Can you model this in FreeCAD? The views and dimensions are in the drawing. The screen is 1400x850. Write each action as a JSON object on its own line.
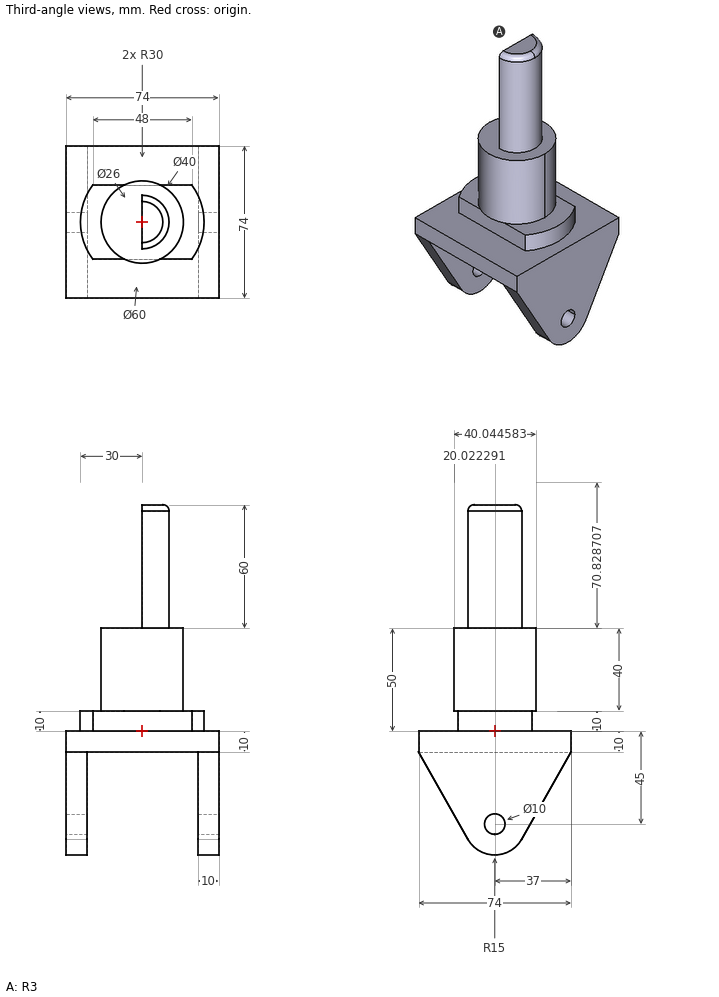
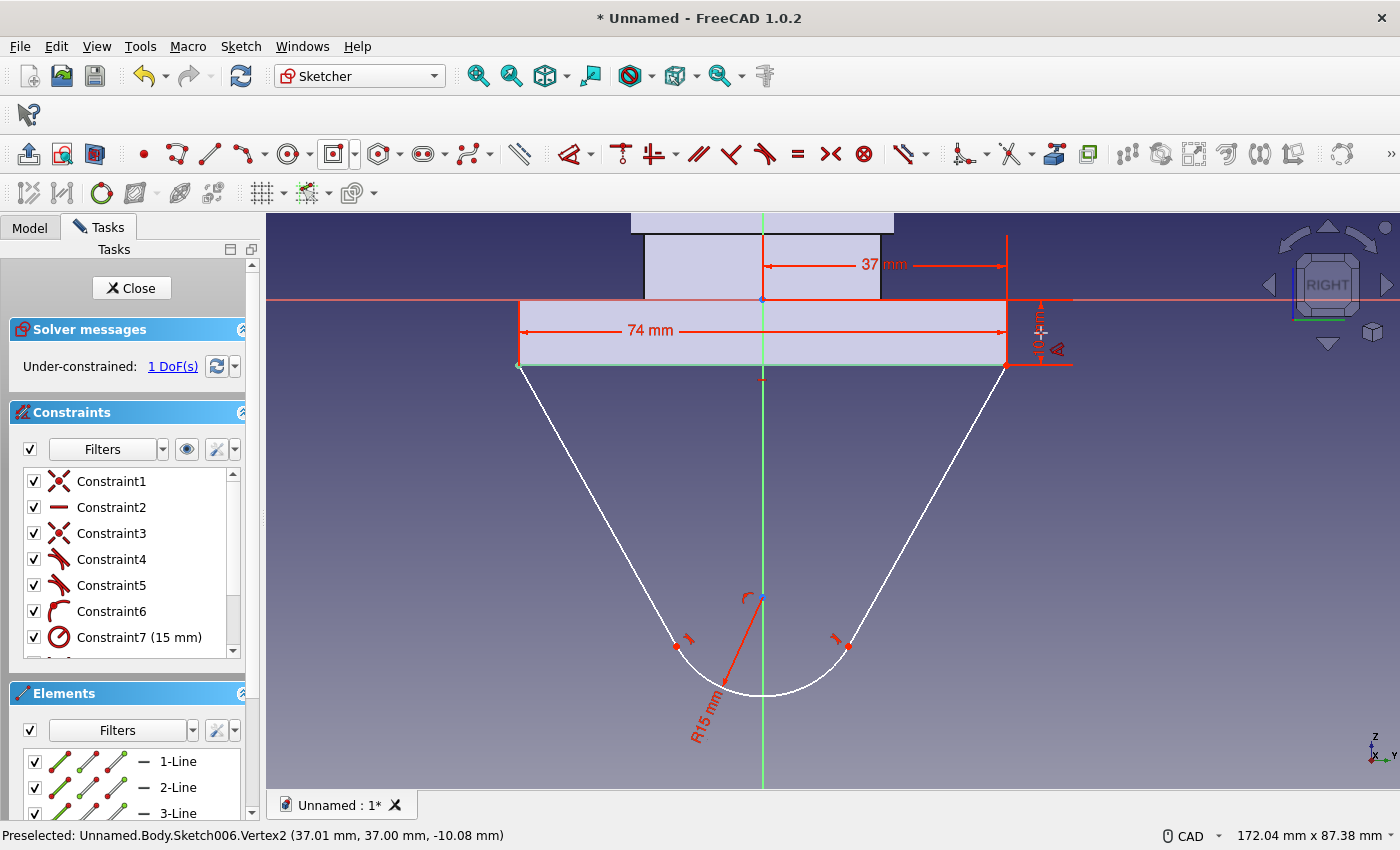
{"action": "left_click", "coordinate": [763, 598]}
{"action": "left_click", "coordinate": [797, 449]}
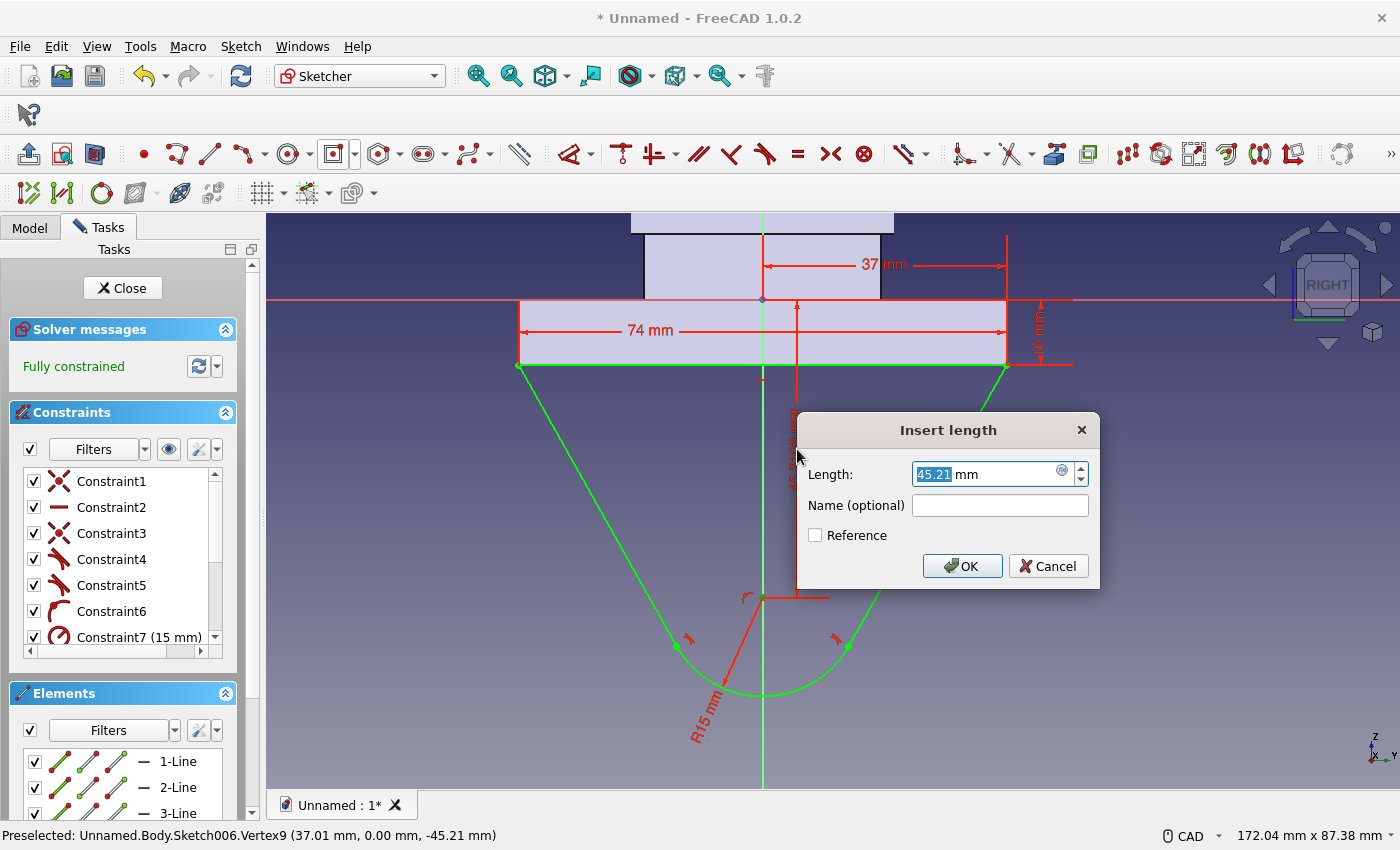
{"action": "type", "text": "45"}
{"action": "key", "text": "Return"}
{"action": "key", "text": "Escape"}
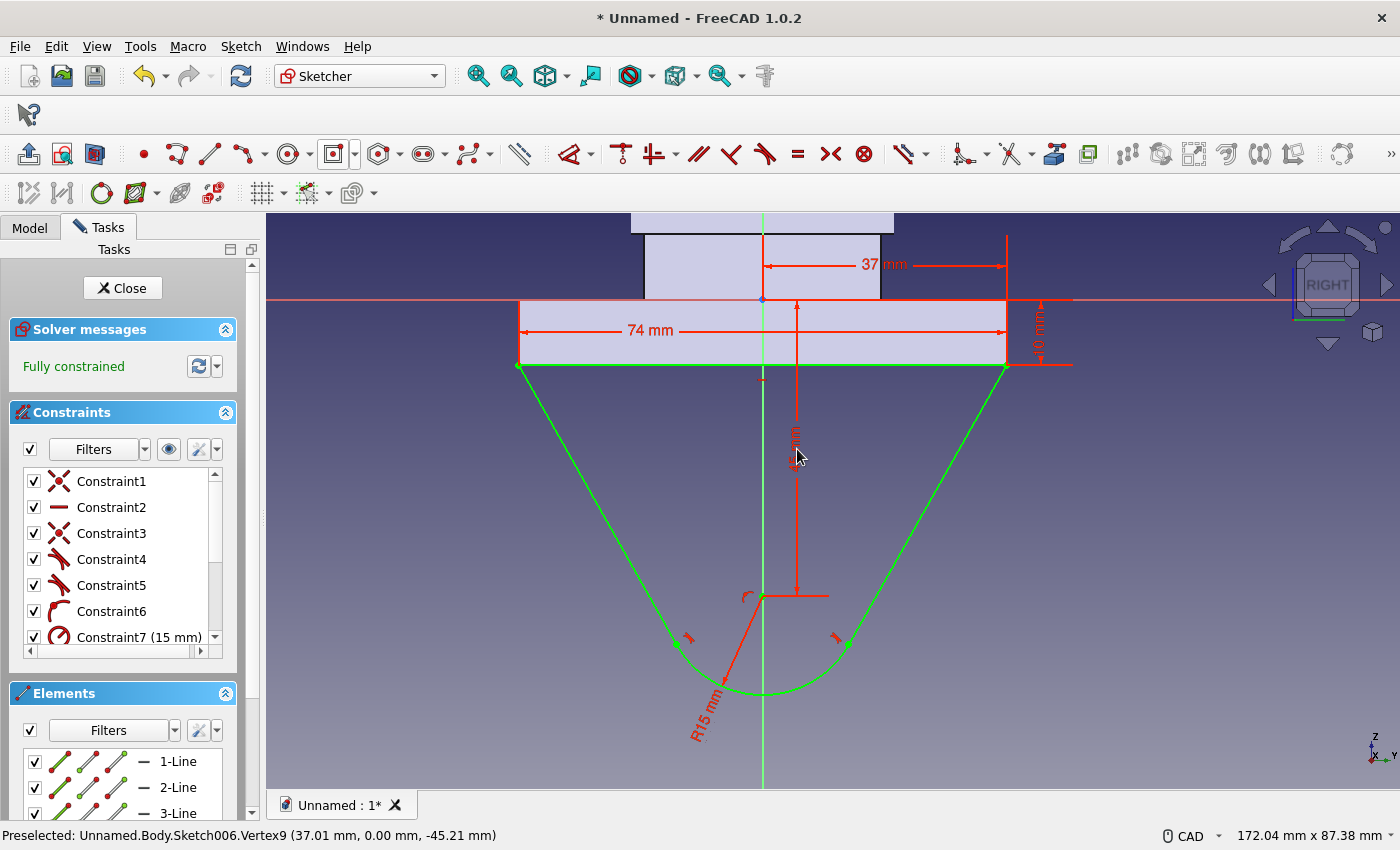
{"action": "left_click", "coordinate": [123, 288]}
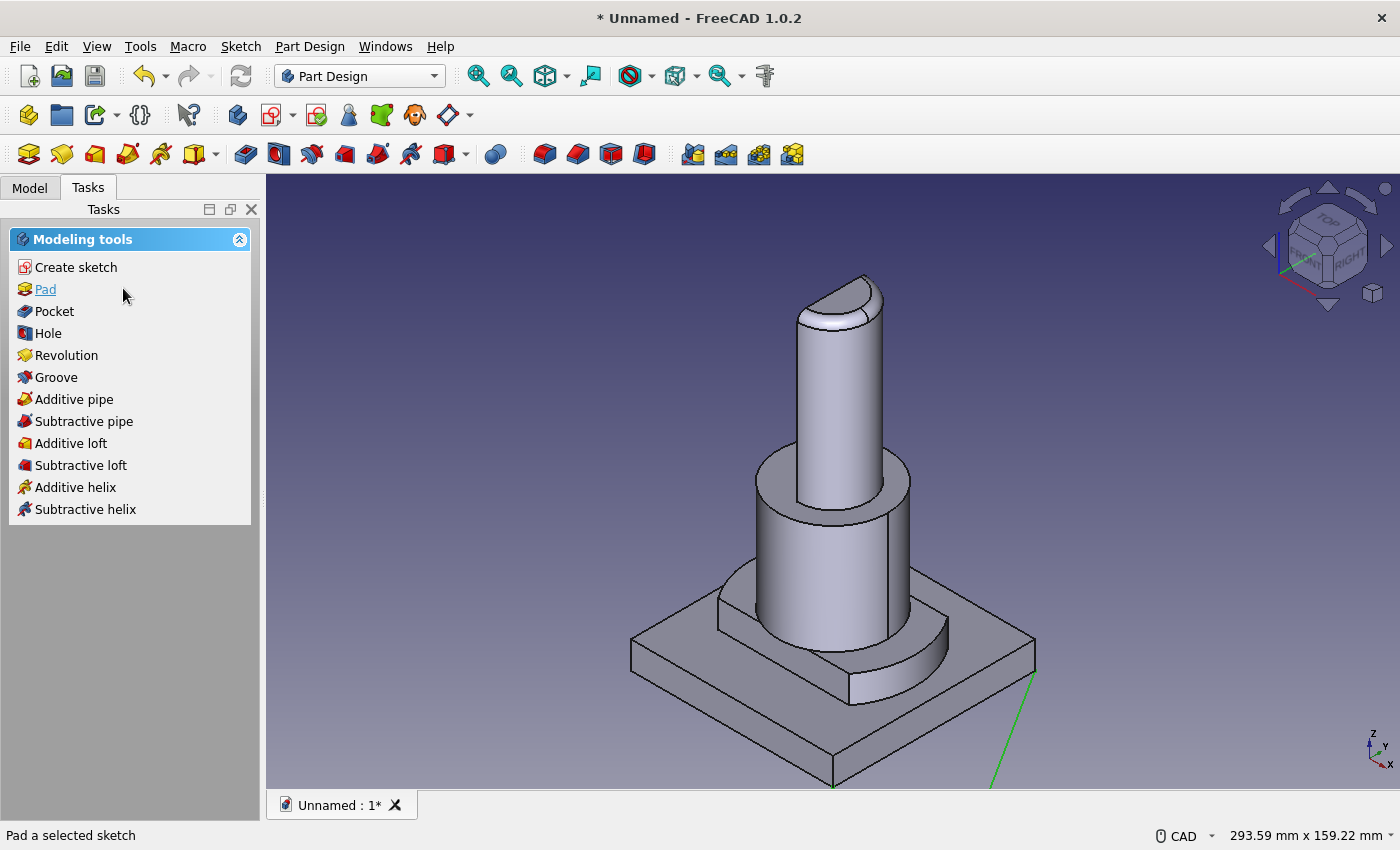
{"action": "left_click", "coordinate": [29, 154]}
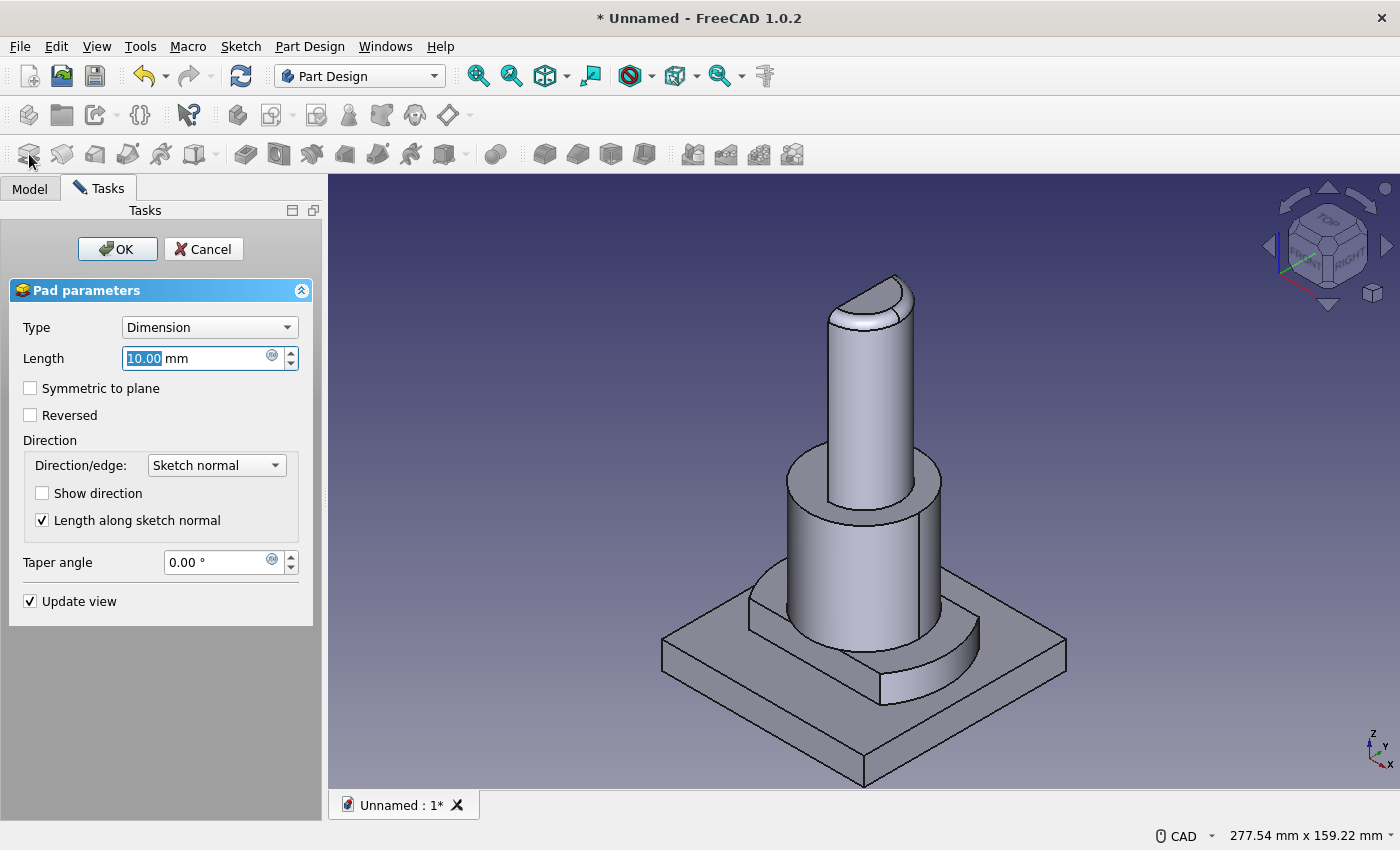
{"action": "type", "text": "10"}
{"action": "key", "text": "Tab"}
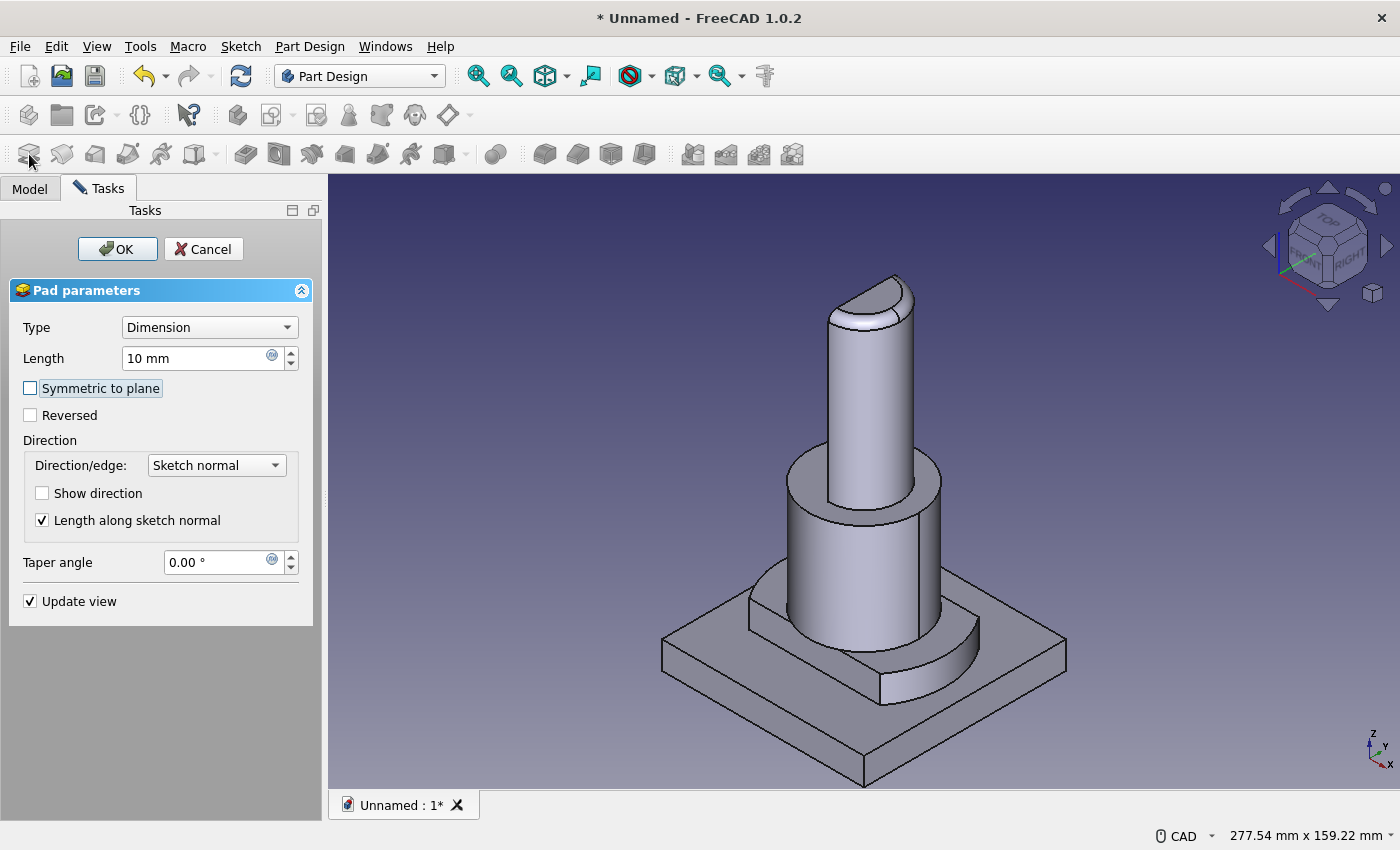
{"action": "left_click", "coordinate": [31, 415]}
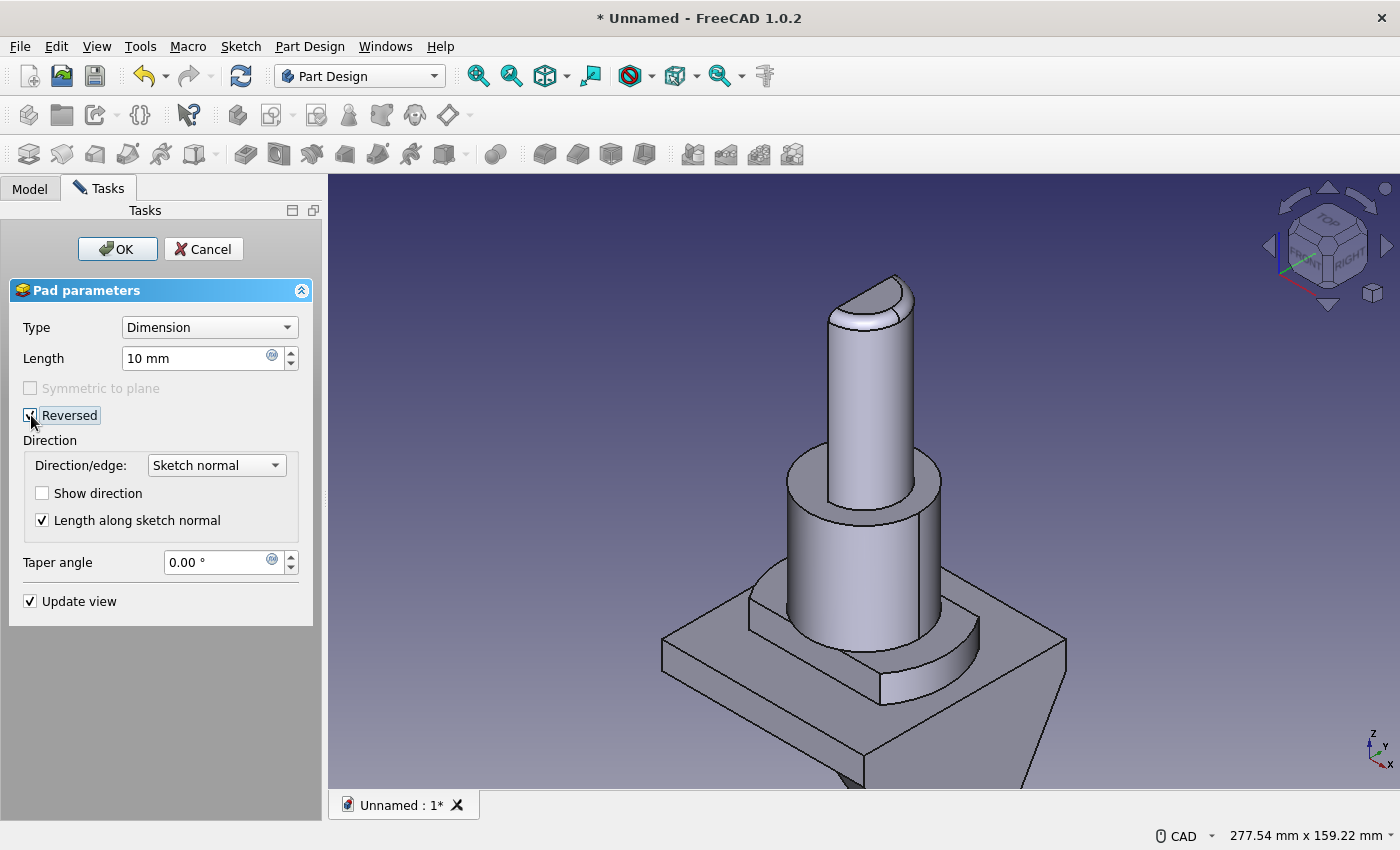
{"action": "left_click", "coordinate": [118, 249]}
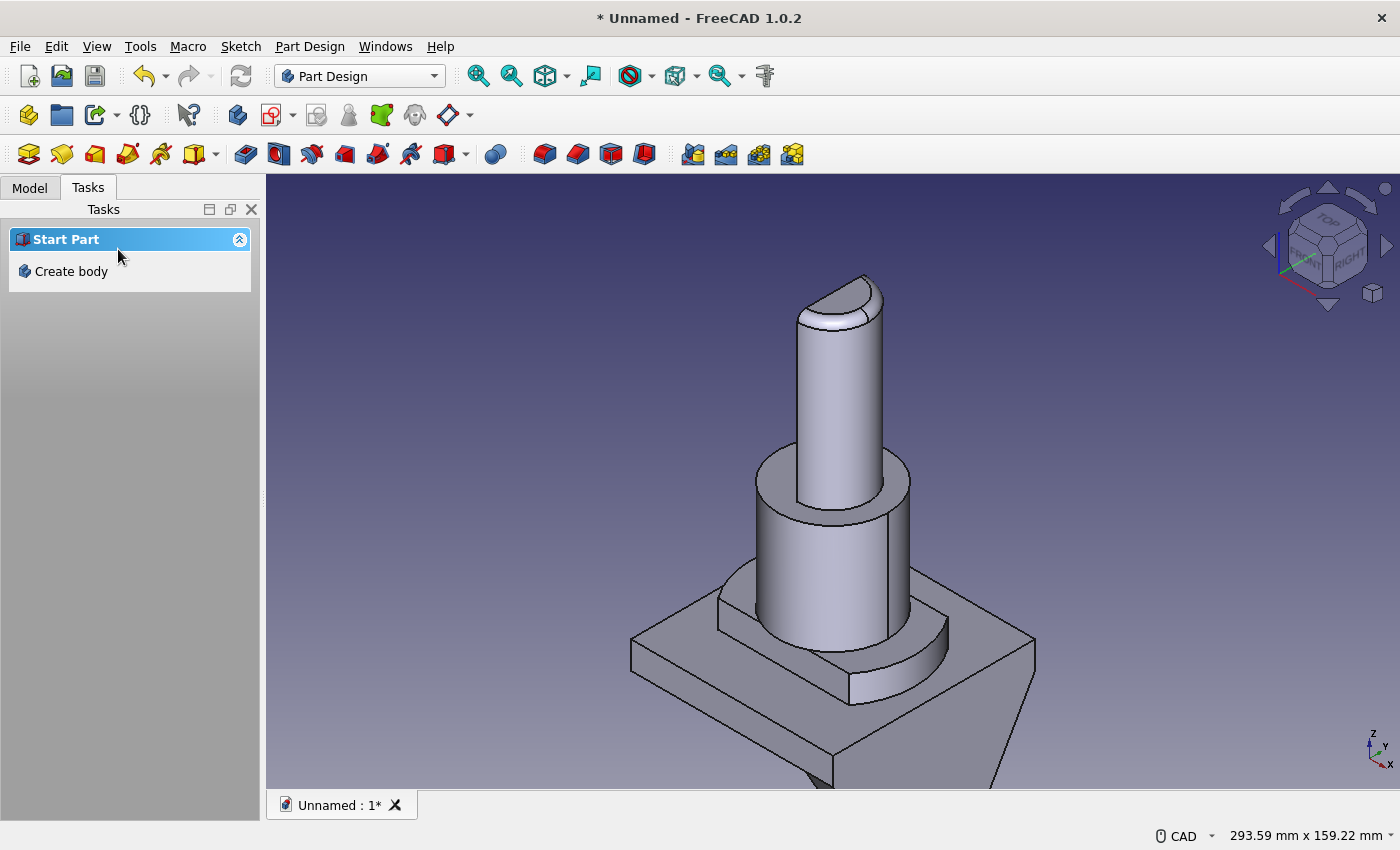
{"action": "left_click", "coordinate": [479, 76]}